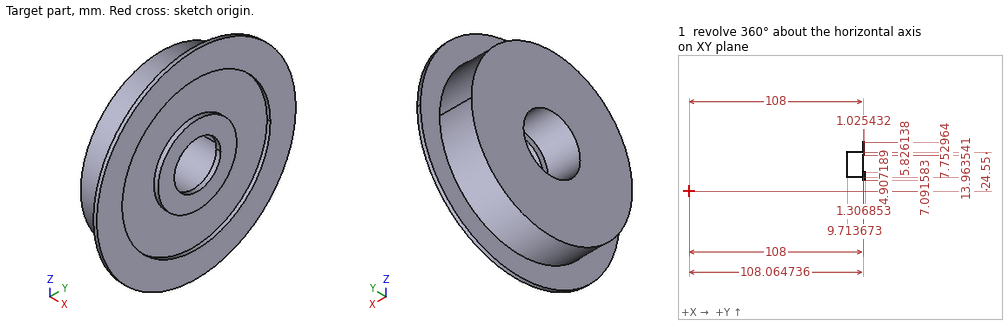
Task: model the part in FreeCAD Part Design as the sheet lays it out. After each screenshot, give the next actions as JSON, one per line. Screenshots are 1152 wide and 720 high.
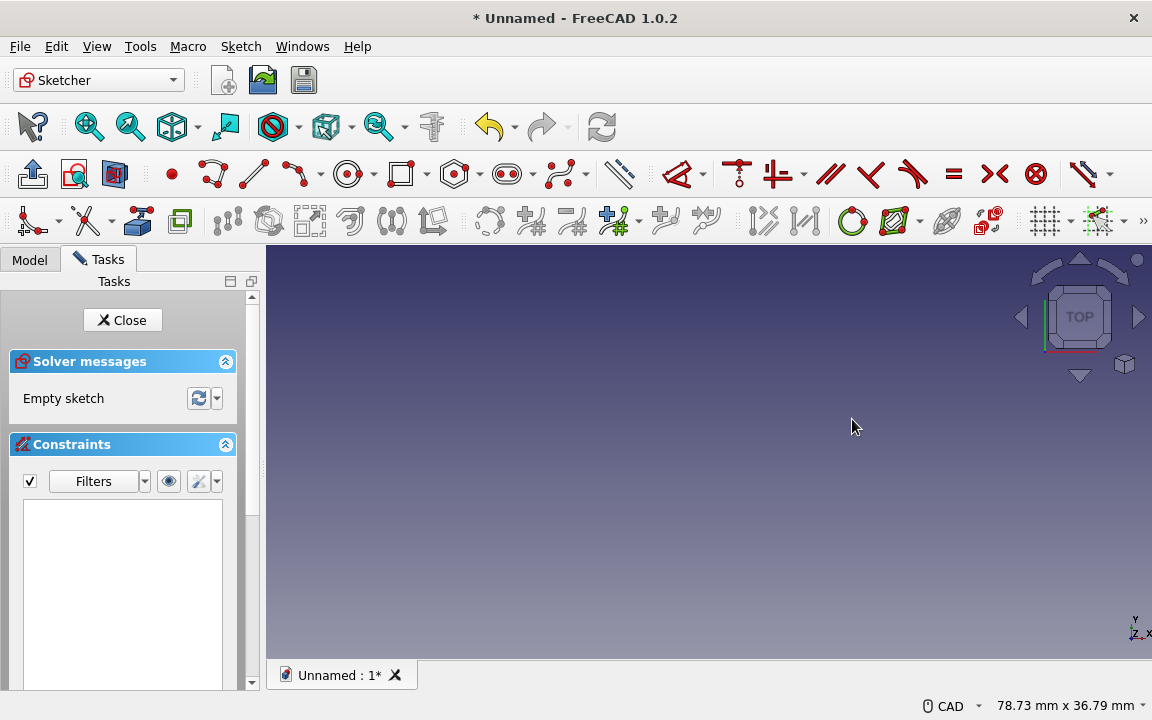
{"action": "left_click", "coordinate": [213, 174]}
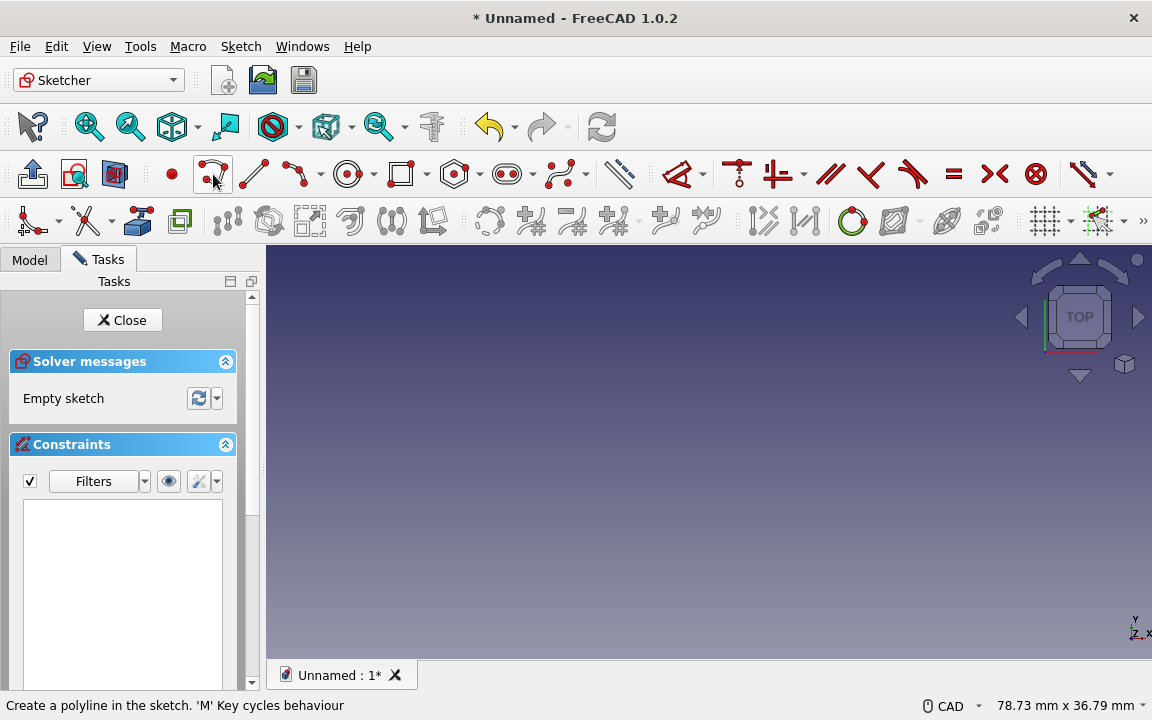
{"action": "left_click", "coordinate": [577, 565]}
{"action": "left_click", "coordinate": [686, 565]}
{"action": "left_click", "coordinate": [686, 408]}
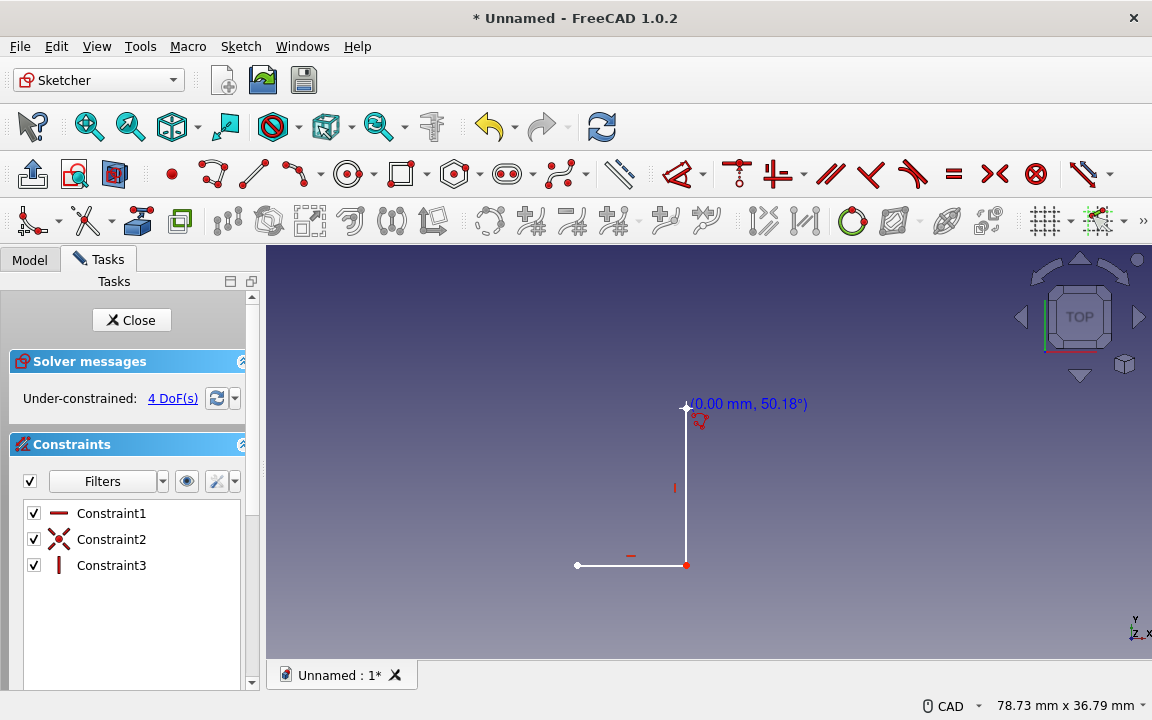
{"action": "scroll", "coordinate": [698, 408], "scroll_direction": "up", "scroll_amount": 2}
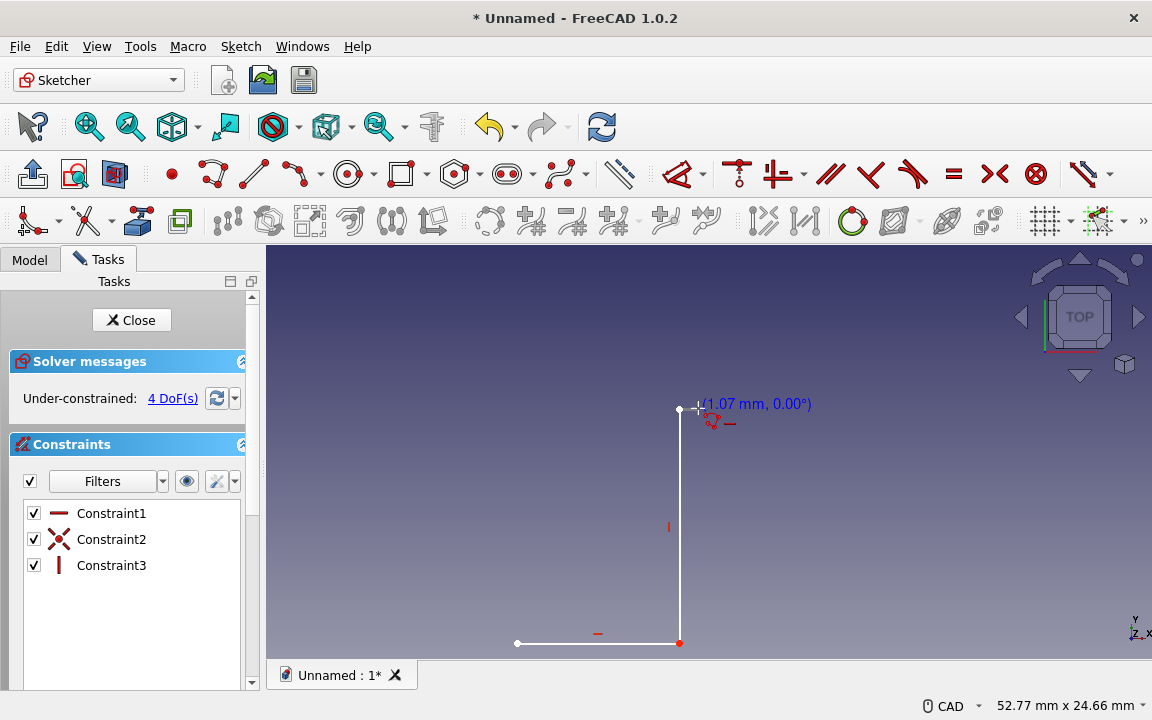
{"action": "left_click", "coordinate": [697, 408]}
{"action": "left_click", "coordinate": [697, 277]}
{"action": "left_click", "coordinate": [680, 277]}
{"action": "left_click", "coordinate": [680, 375]}
{"action": "left_click", "coordinate": [517, 375]}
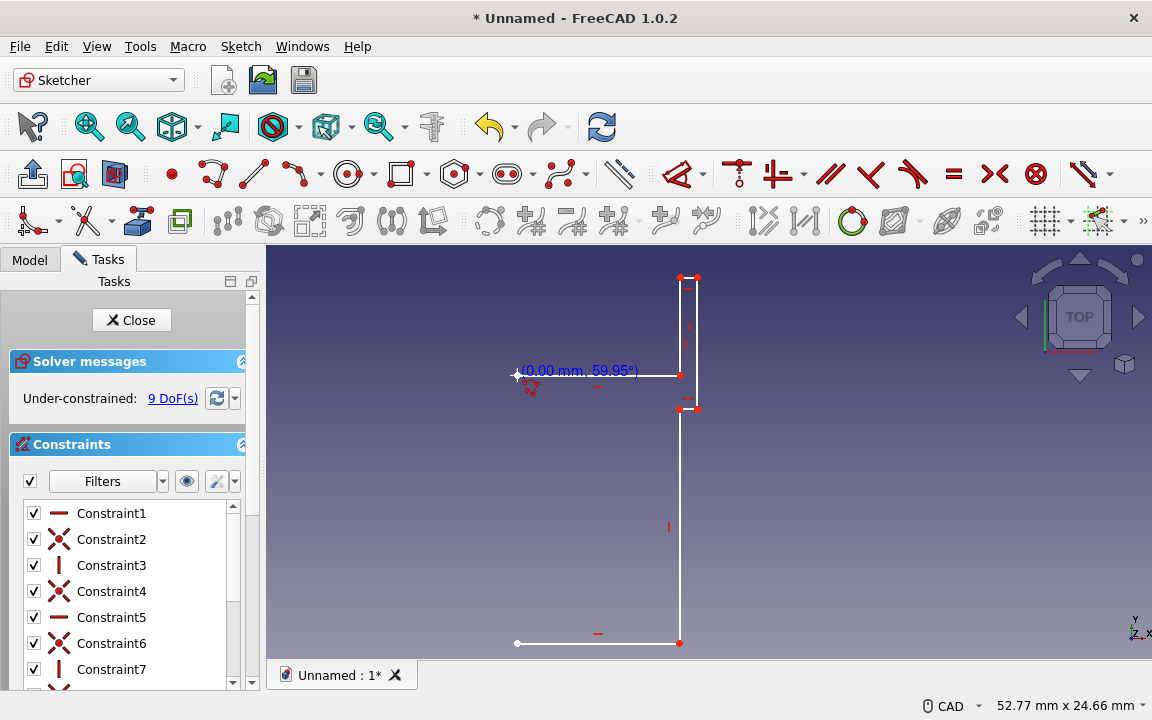
{"action": "scroll", "coordinate": [702, 409], "scroll_direction": "down", "scroll_amount": 2}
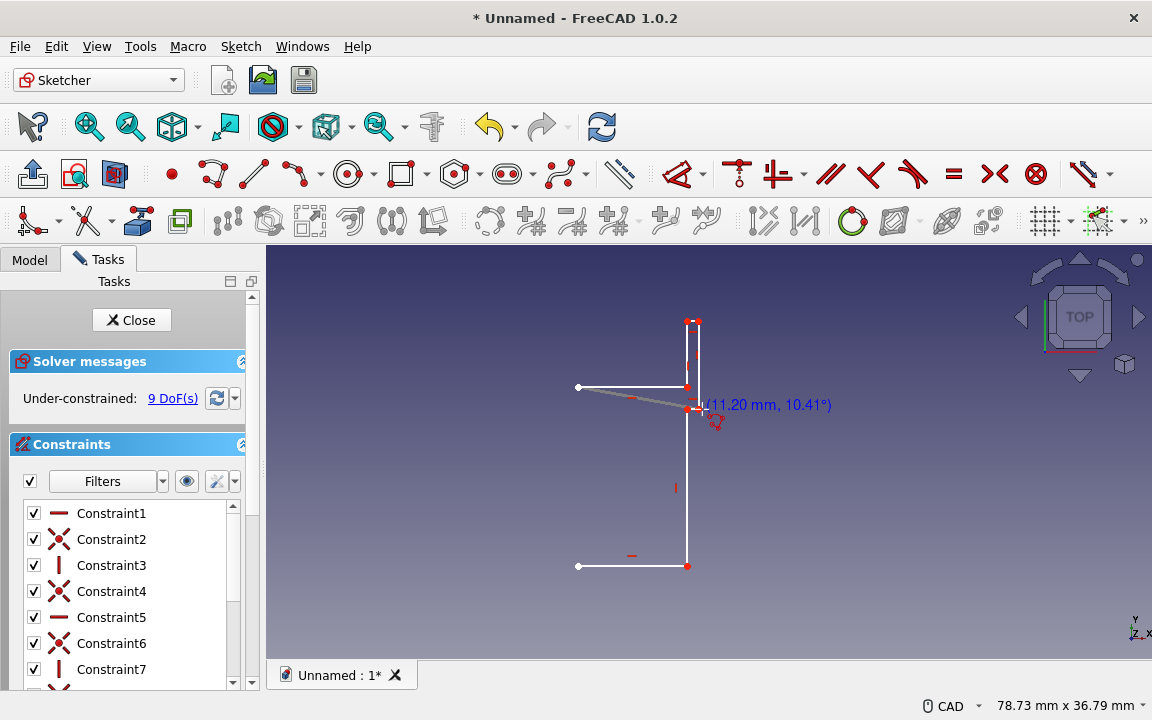
{"action": "left_click", "coordinate": [578, 566]}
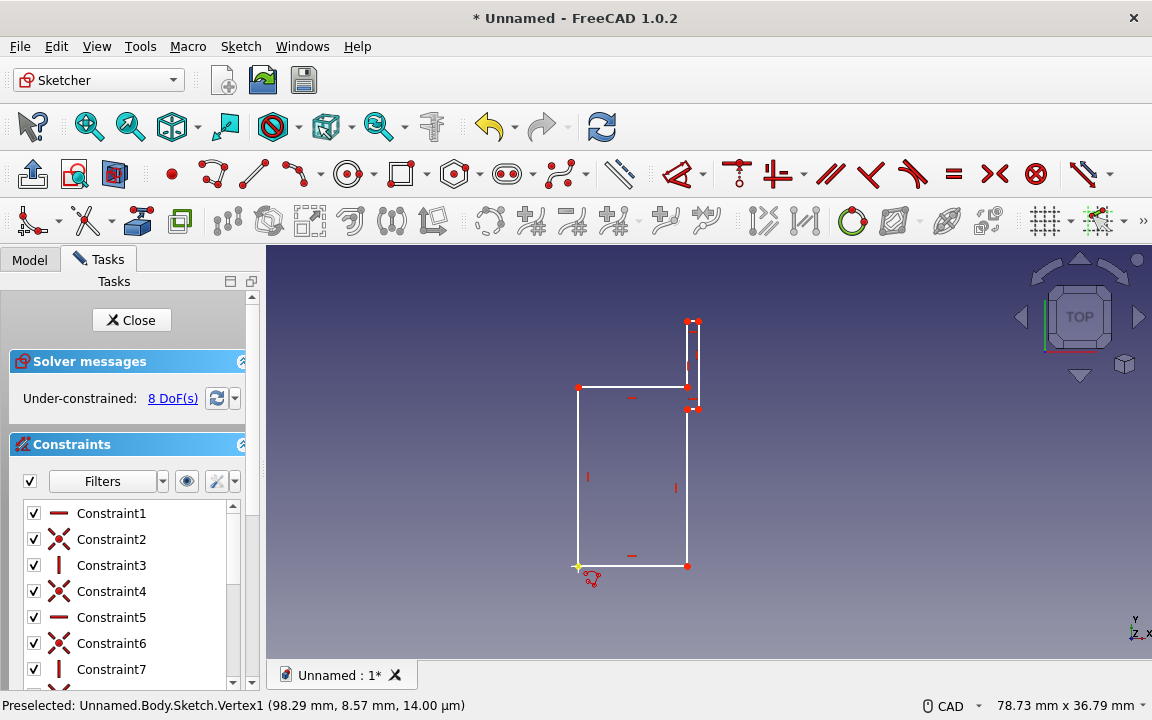
{"action": "left_click", "coordinate": [400, 174]}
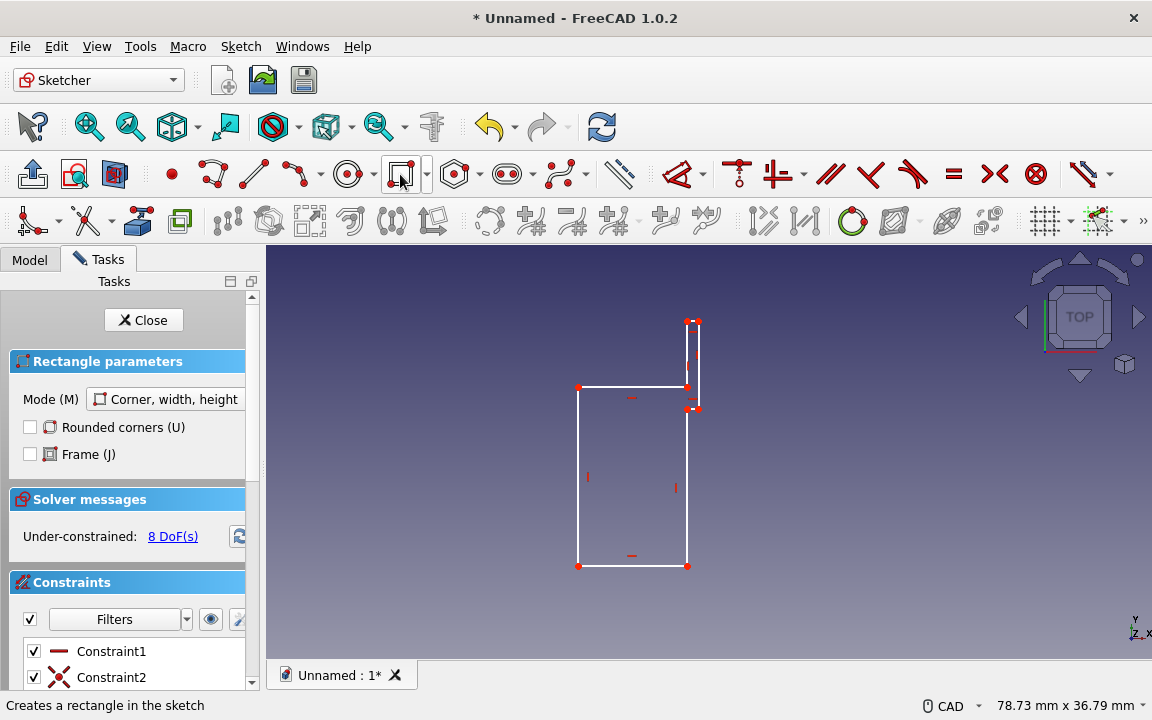
{"action": "scroll", "coordinate": [688, 528], "scroll_direction": "up", "scroll_amount": 16}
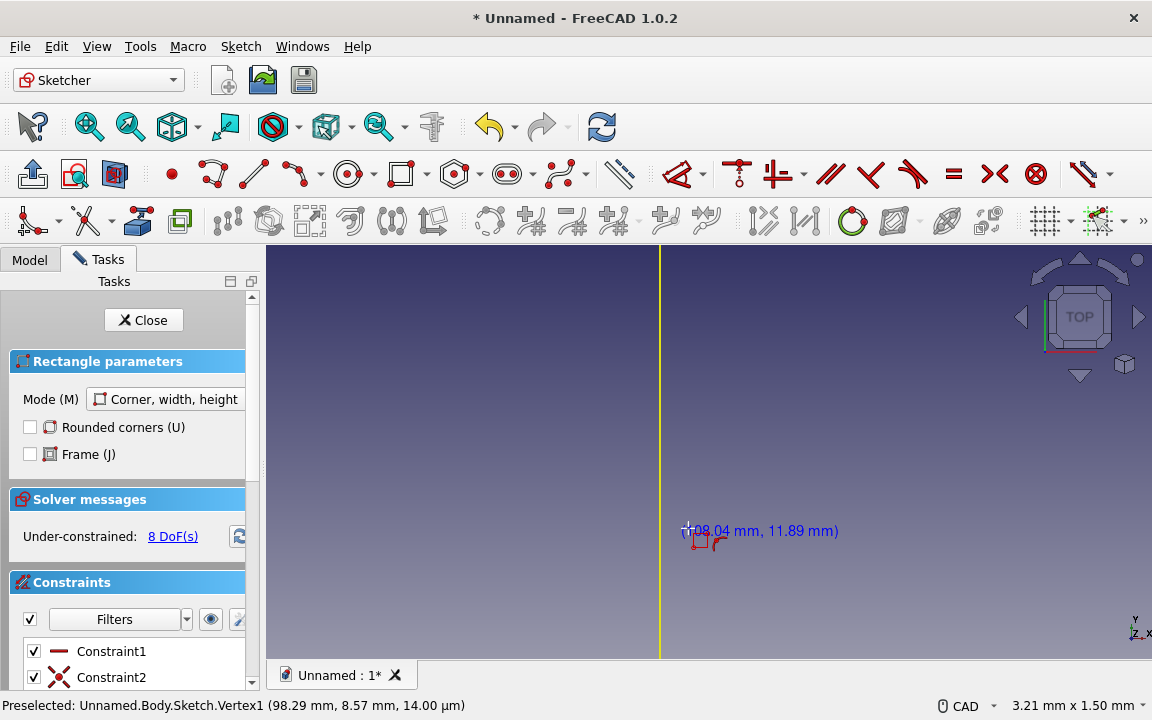
{"action": "left_click", "coordinate": [683, 507]}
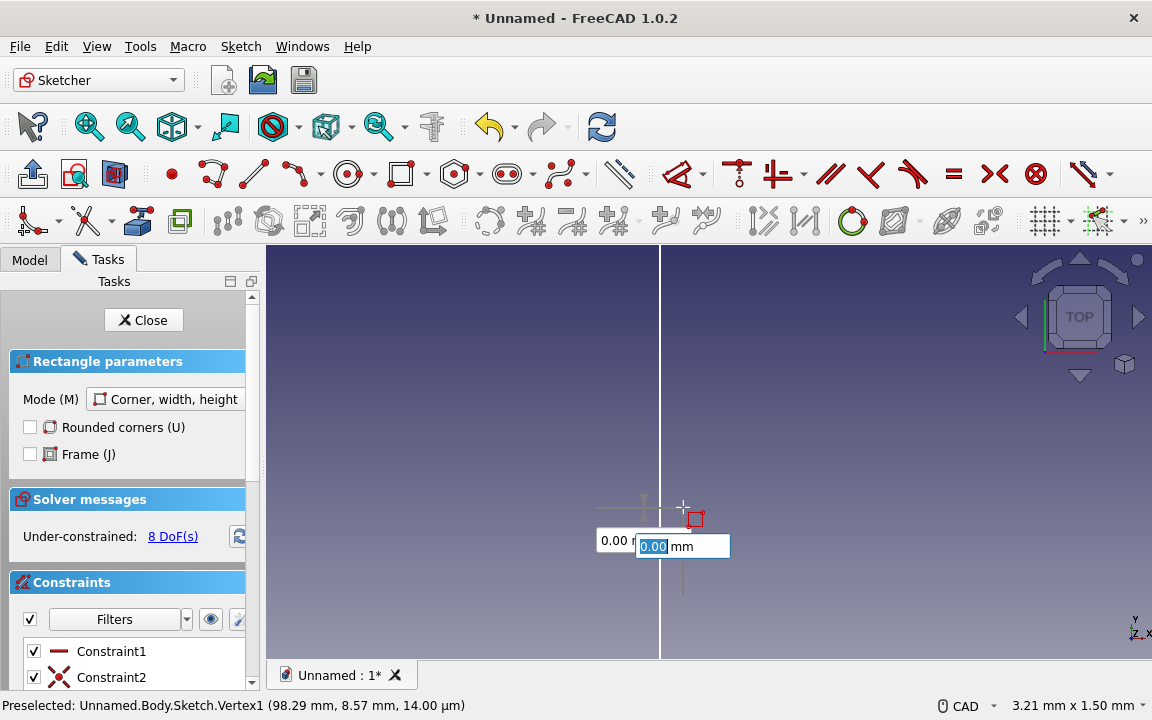
{"action": "scroll", "coordinate": [688, 529], "scroll_direction": "down", "scroll_amount": 16}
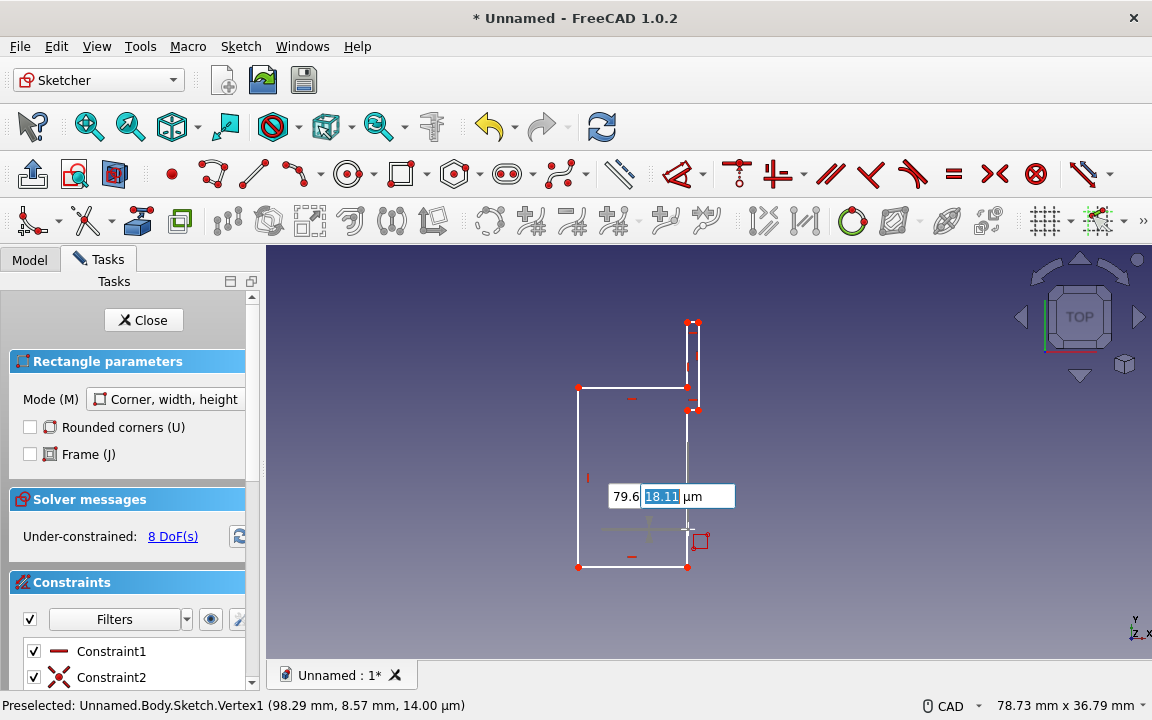
{"action": "left_click", "coordinate": [703, 584]}
{"action": "key", "text": "Escape"}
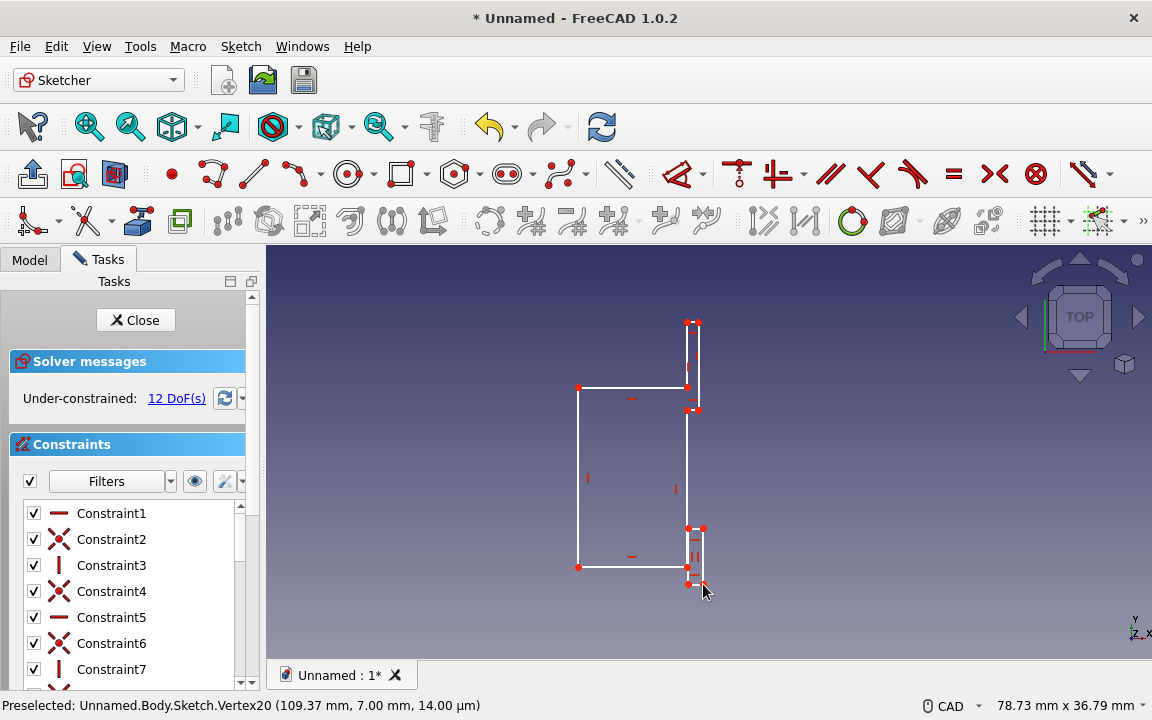
{"action": "left_click", "coordinate": [676, 174]}